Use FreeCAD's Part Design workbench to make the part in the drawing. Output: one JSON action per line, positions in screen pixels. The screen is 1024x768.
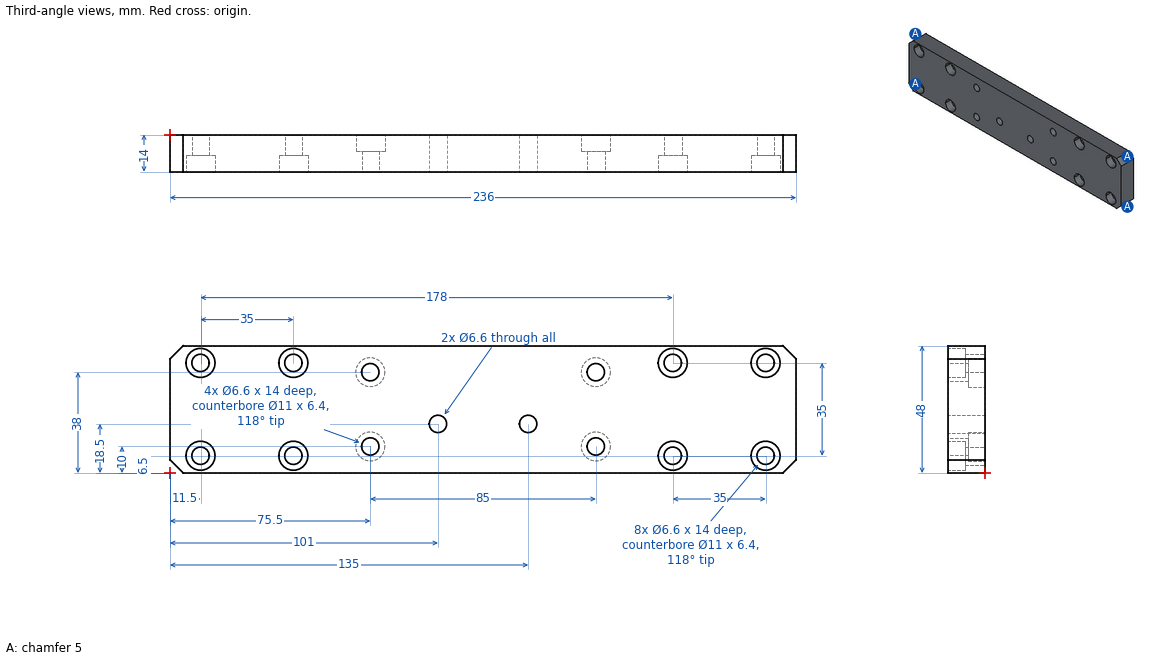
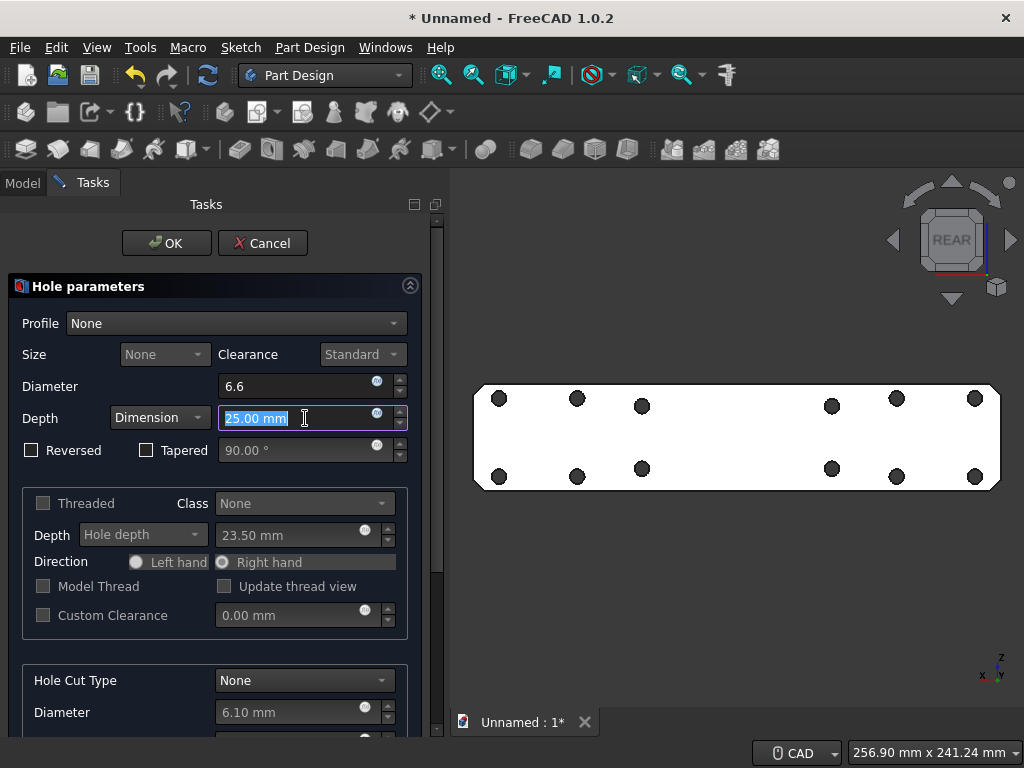
{"action": "type", "text": "14"}
{"action": "key", "text": "Tab"}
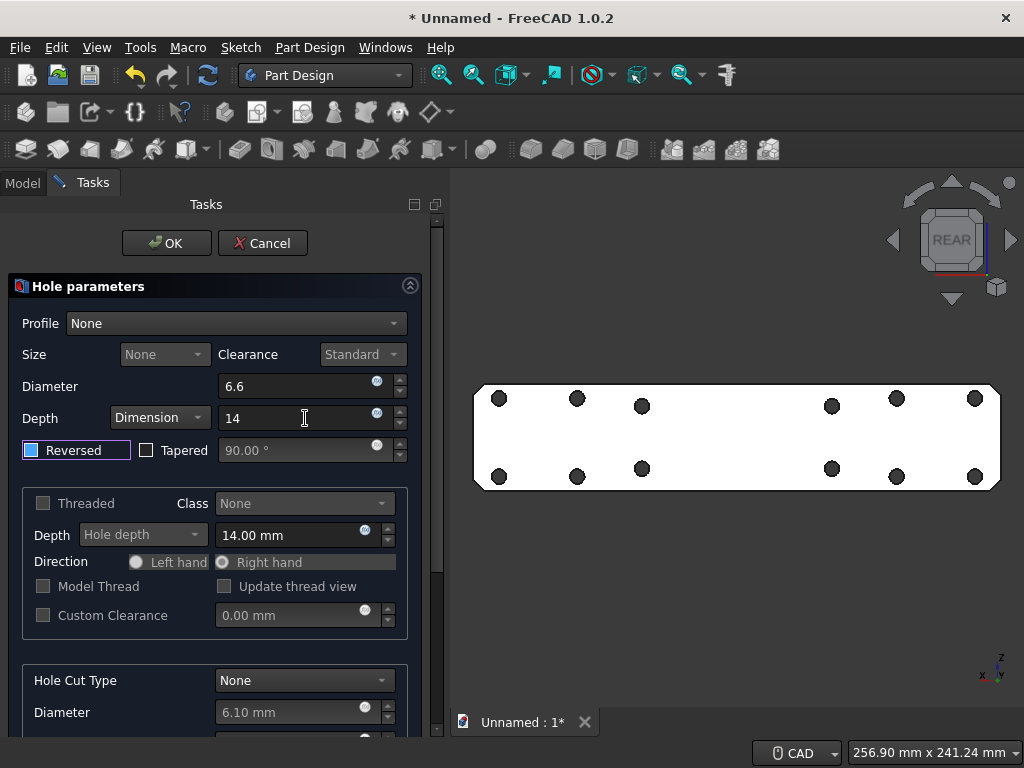
{"action": "left_click", "coordinate": [306, 680]}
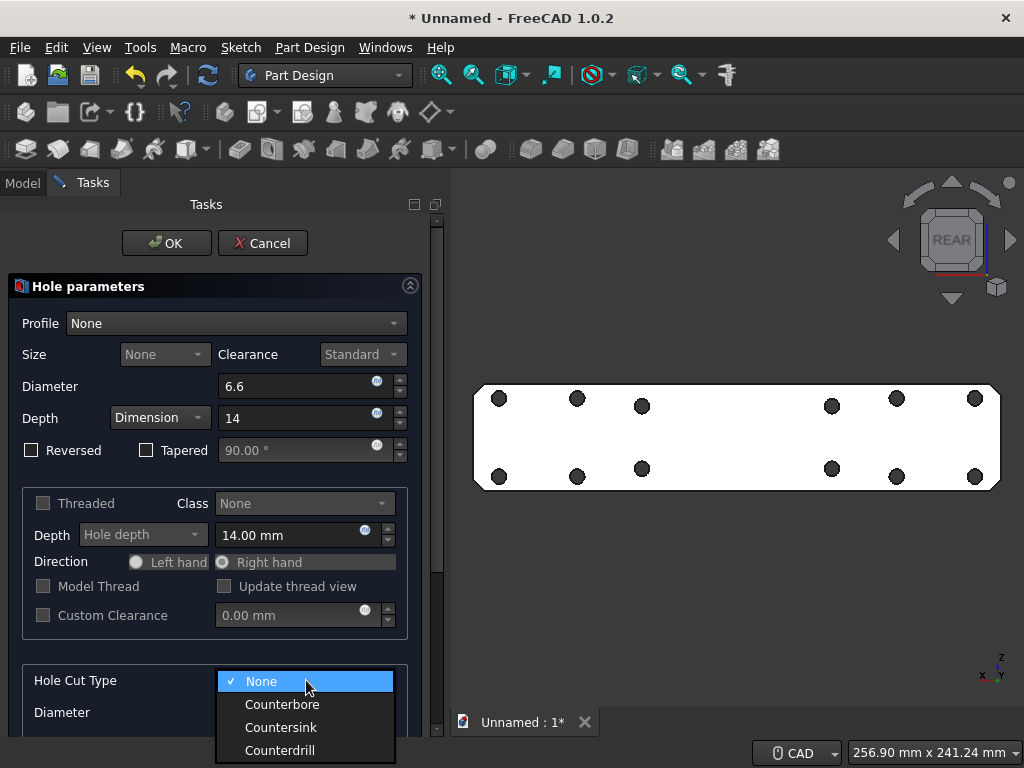
{"action": "left_click", "coordinate": [304, 704]}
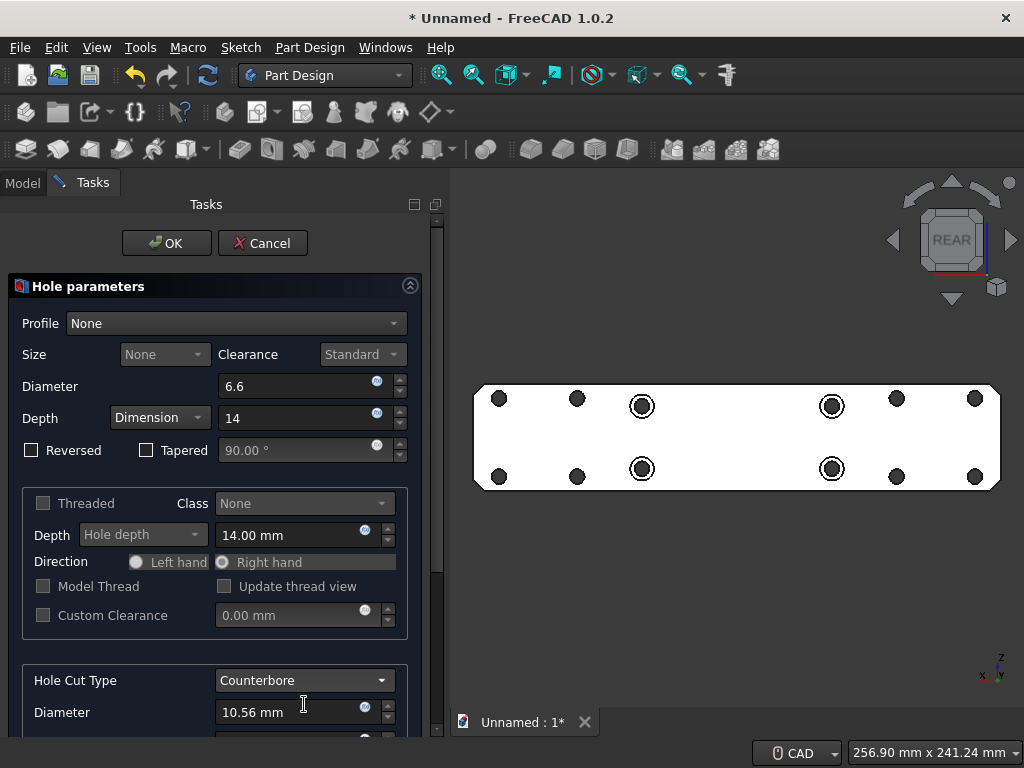
{"action": "triple_click", "coordinate": [298, 712]}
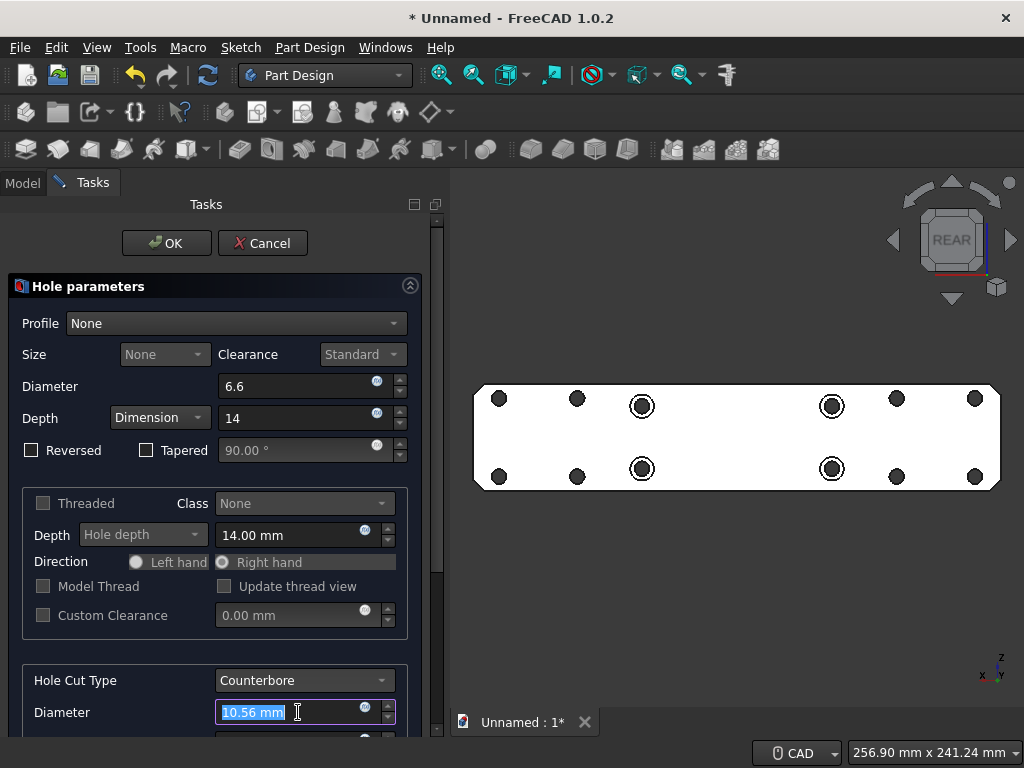
{"action": "type", "text": "11"}
{"action": "key", "text": "Tab"}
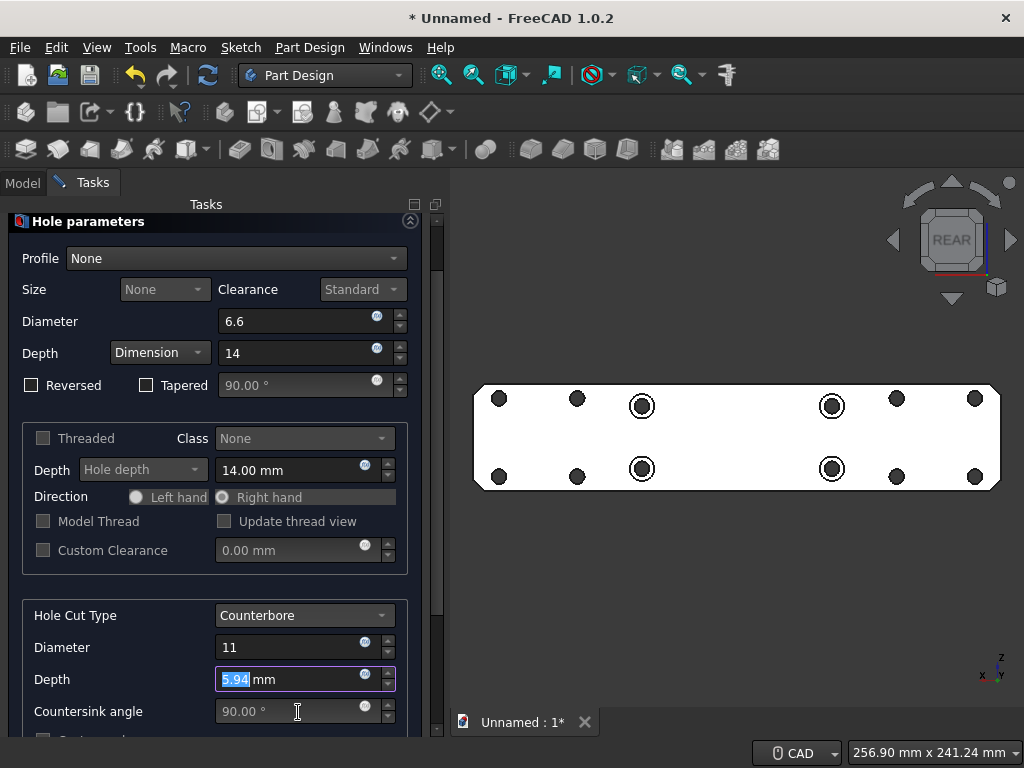
{"action": "type", "text": "6.4"}
{"action": "key", "text": "Tab"}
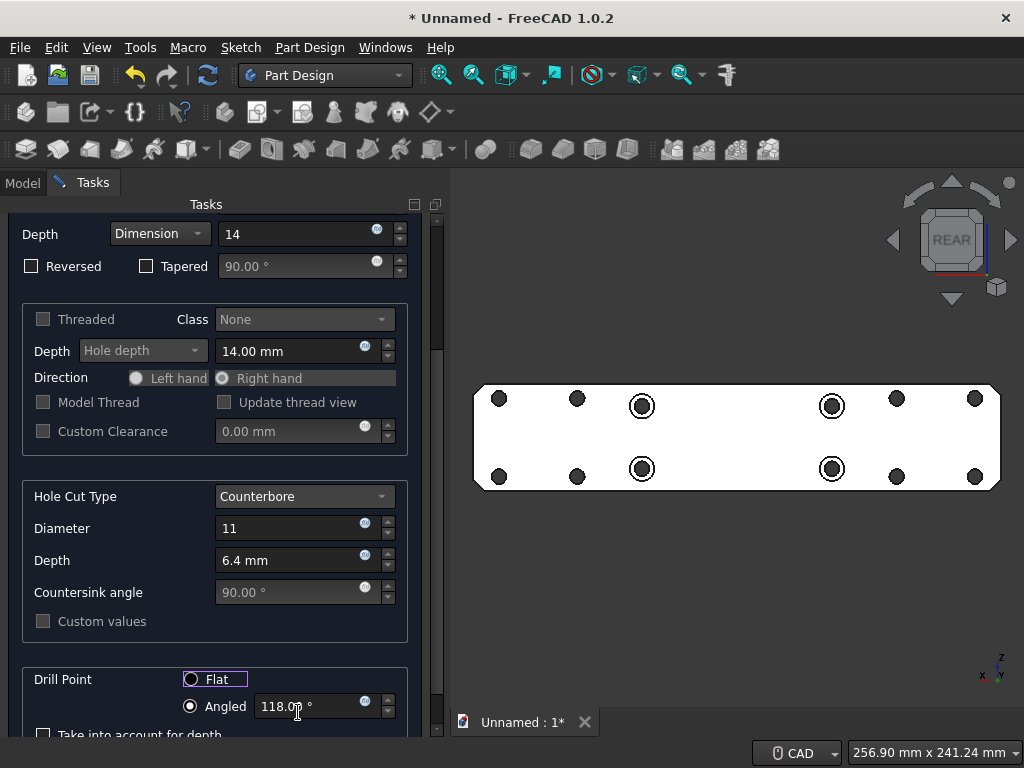
{"action": "scroll", "coordinate": [437, 475], "scroll_direction": "up", "scroll_amount": 4}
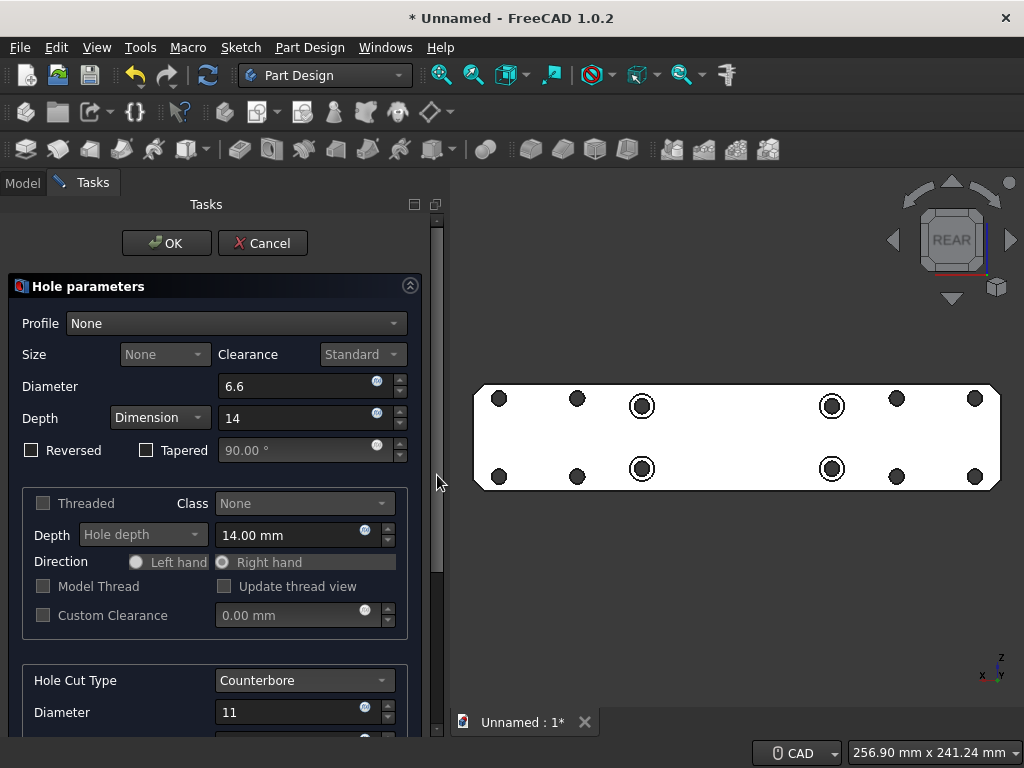
{"action": "left_click", "coordinate": [167, 243]}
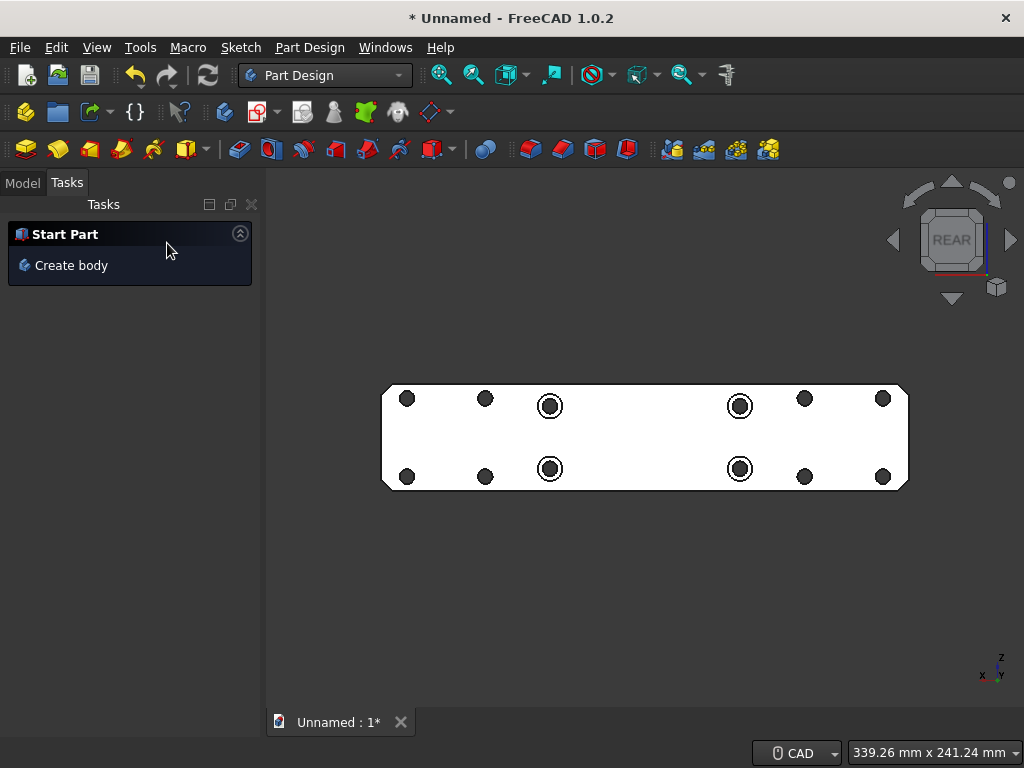
{"action": "left_click", "coordinate": [258, 112]}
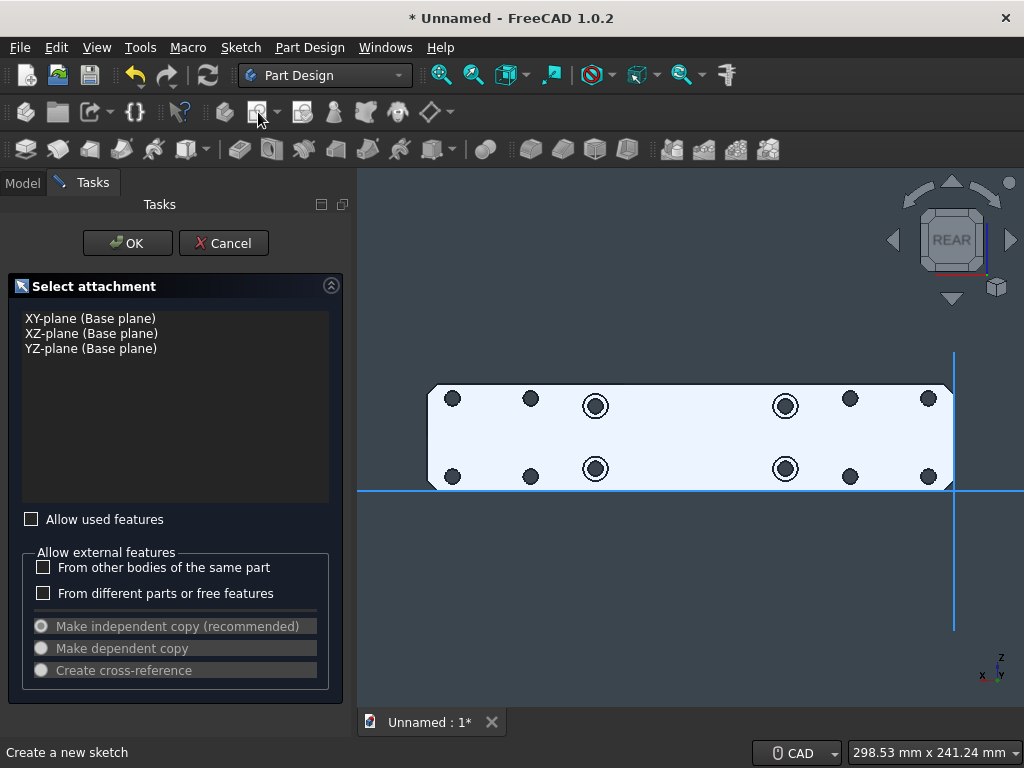
{"action": "left_click", "coordinate": [82, 334]}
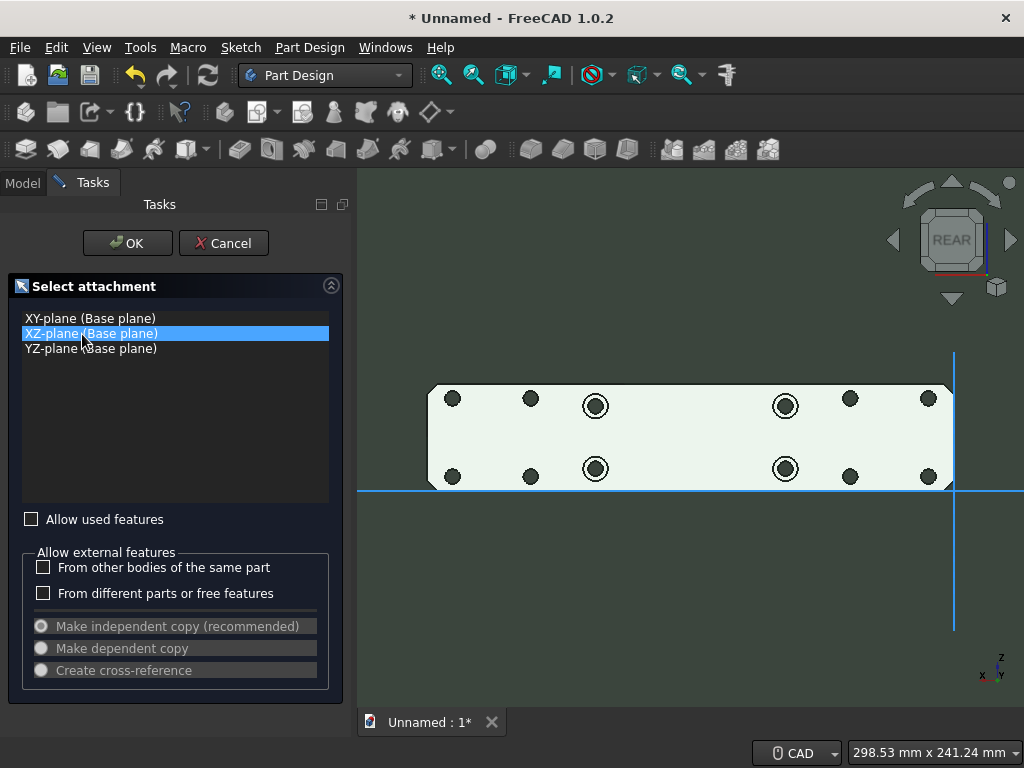
{"action": "left_click", "coordinate": [128, 243]}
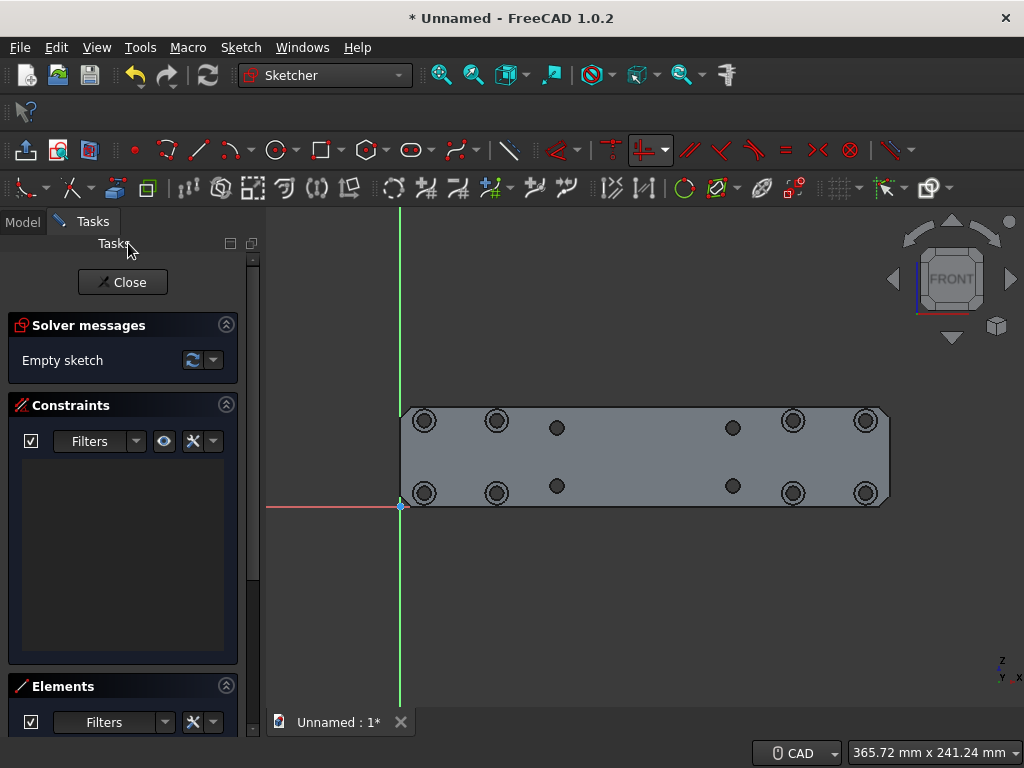
{"action": "left_click", "coordinate": [90, 150]}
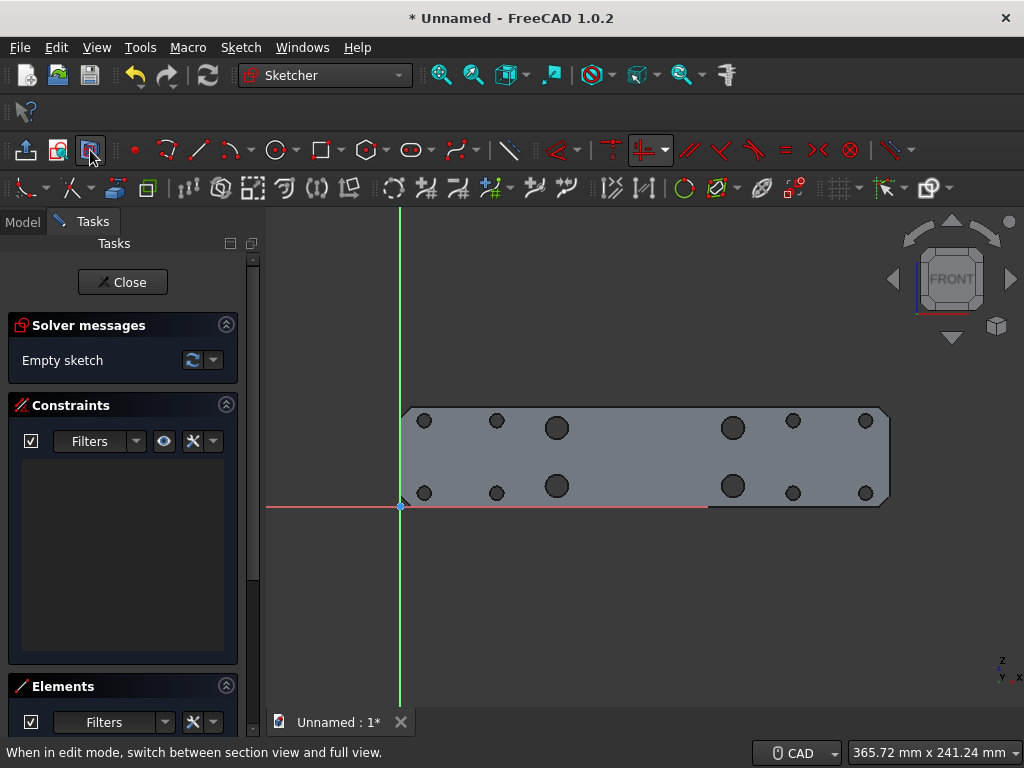
{"action": "scroll", "coordinate": [662, 471], "scroll_direction": "up", "scroll_amount": 8}